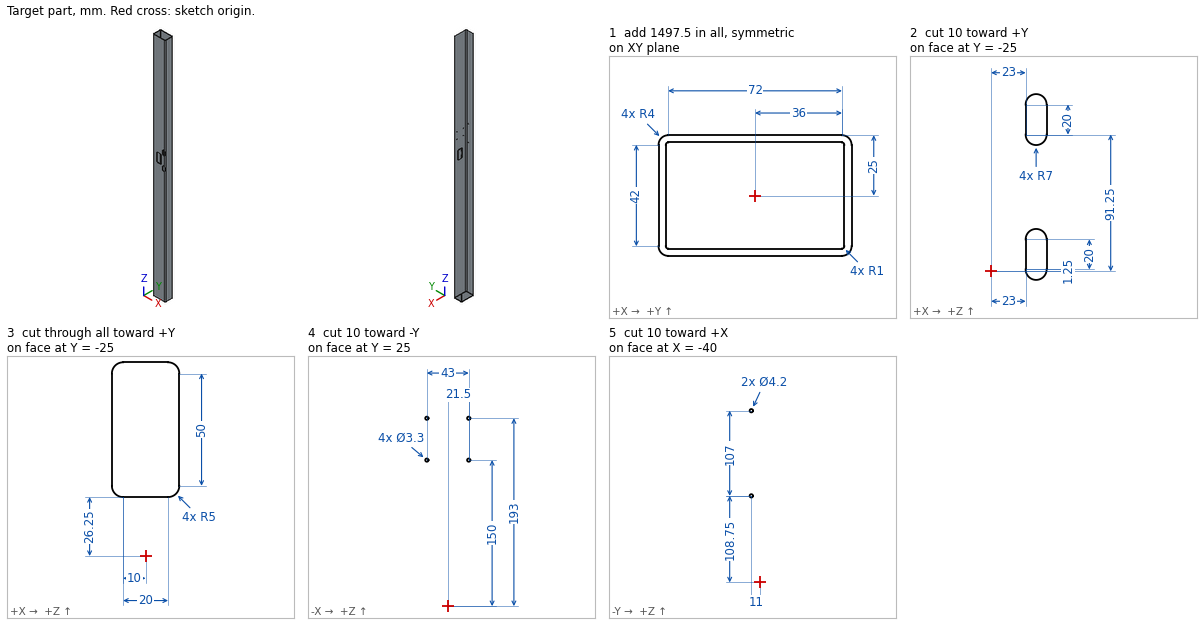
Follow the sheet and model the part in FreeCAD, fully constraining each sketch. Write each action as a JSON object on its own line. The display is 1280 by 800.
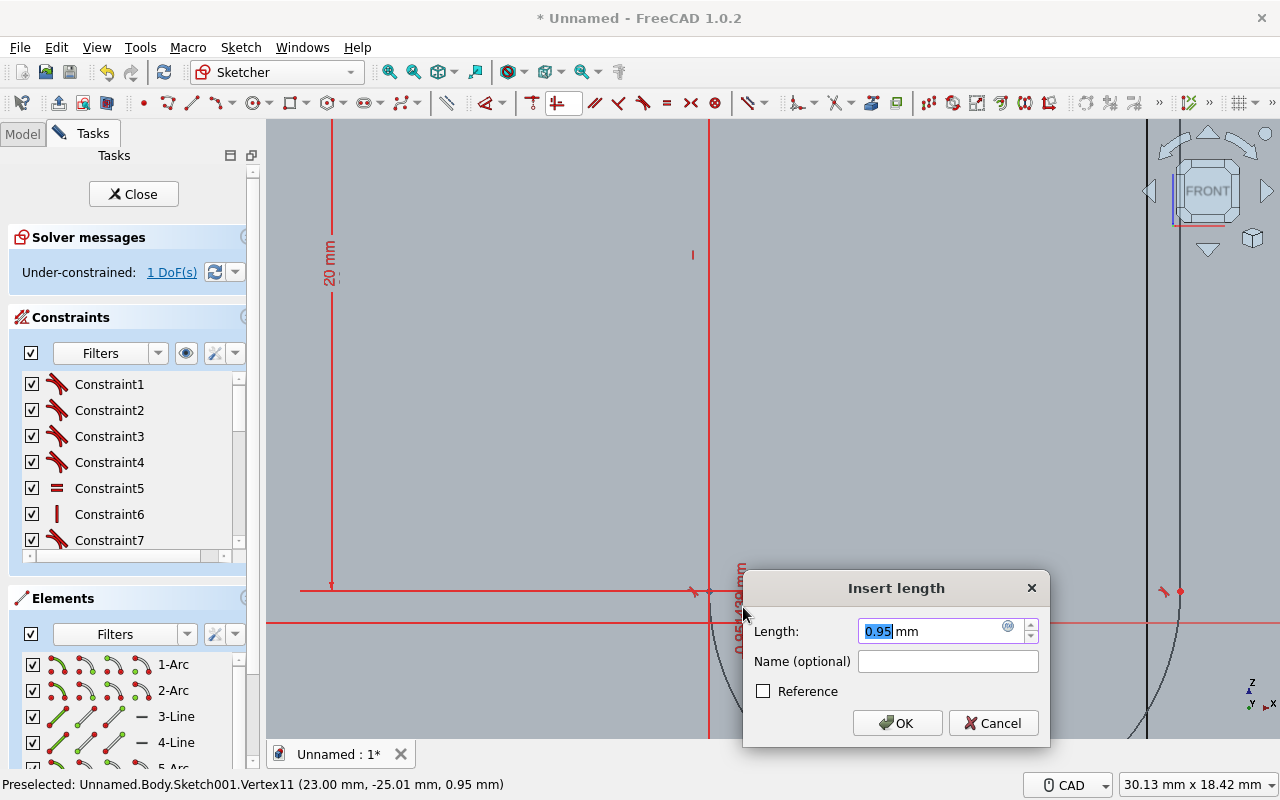
{"action": "type", "text": "1.25"}
{"action": "key", "text": "Return"}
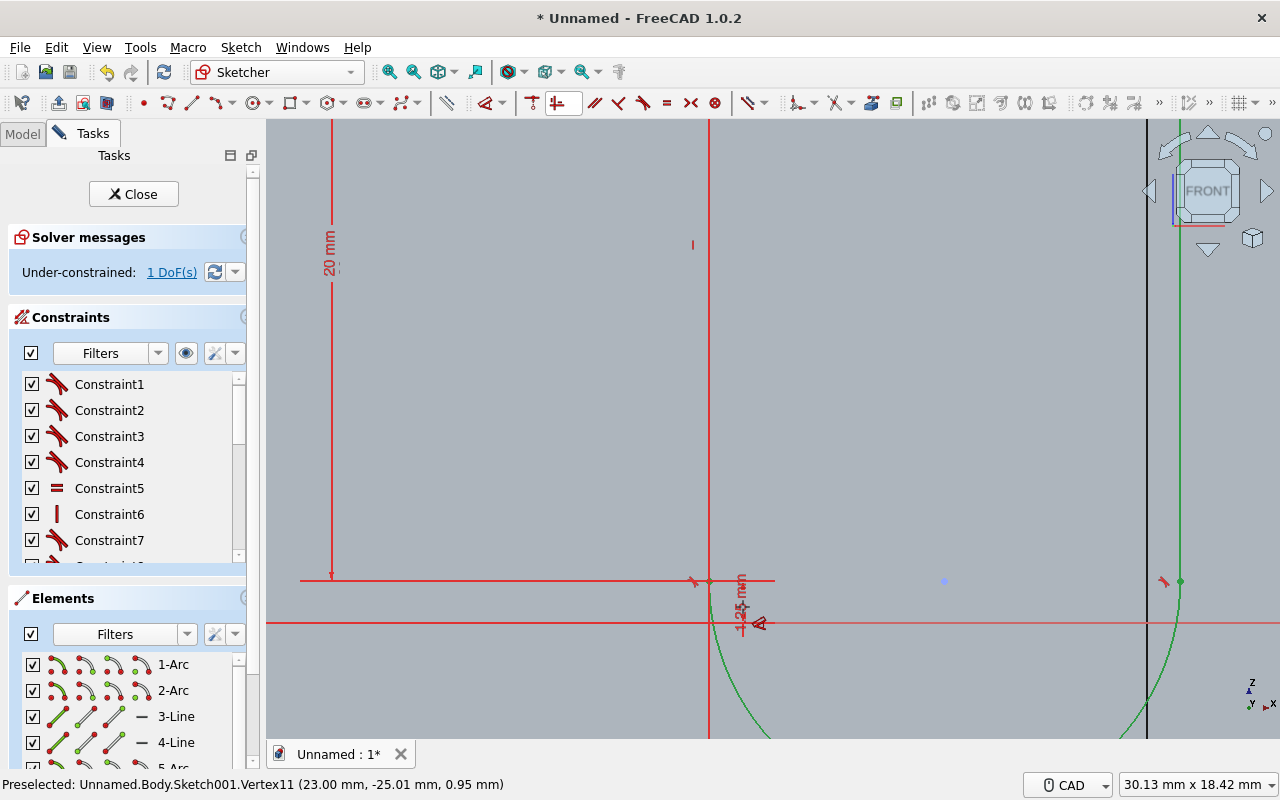
{"action": "scroll", "coordinate": [719, 599], "scroll_direction": "down", "scroll_amount": 12}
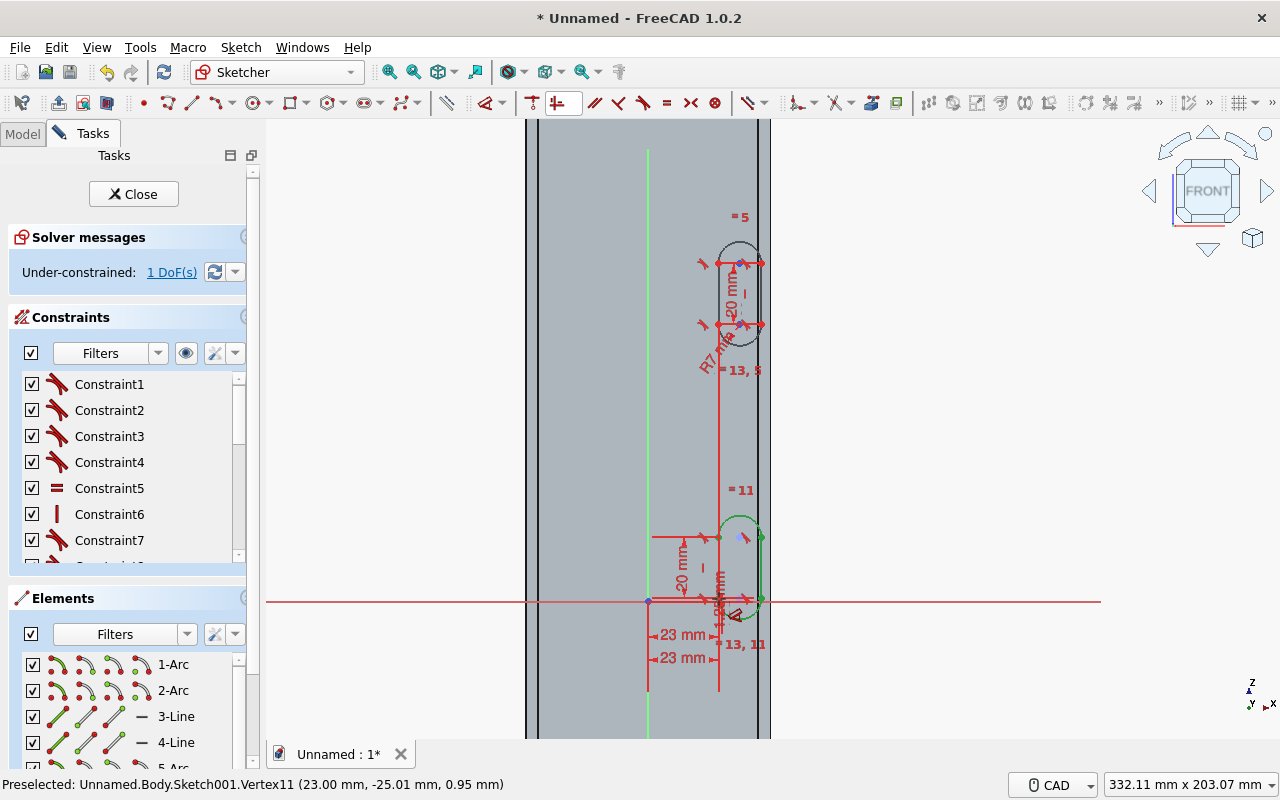
{"action": "left_click", "coordinate": [719, 324]}
{"action": "left_click", "coordinate": [614, 463]}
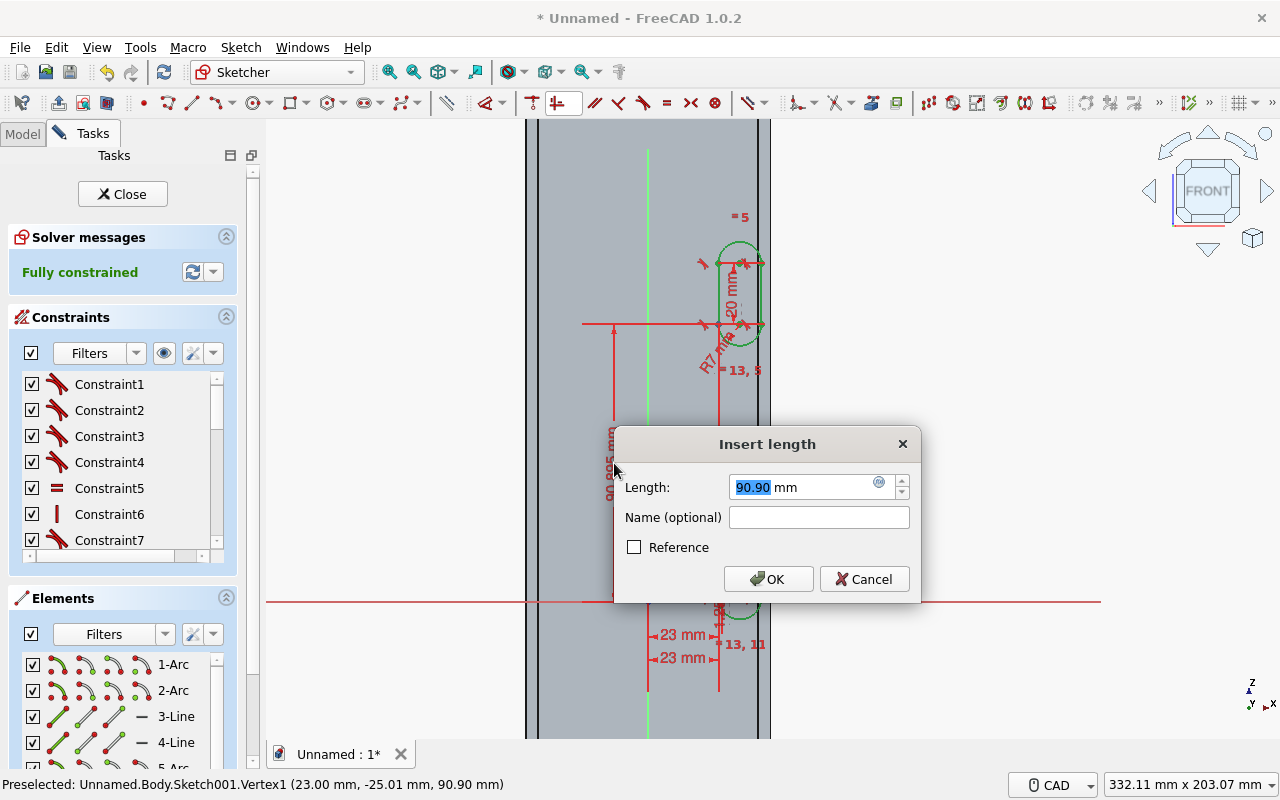
{"action": "type", "text": "91.25"}
{"action": "key", "text": "Return"}
{"action": "key", "text": "Escape"}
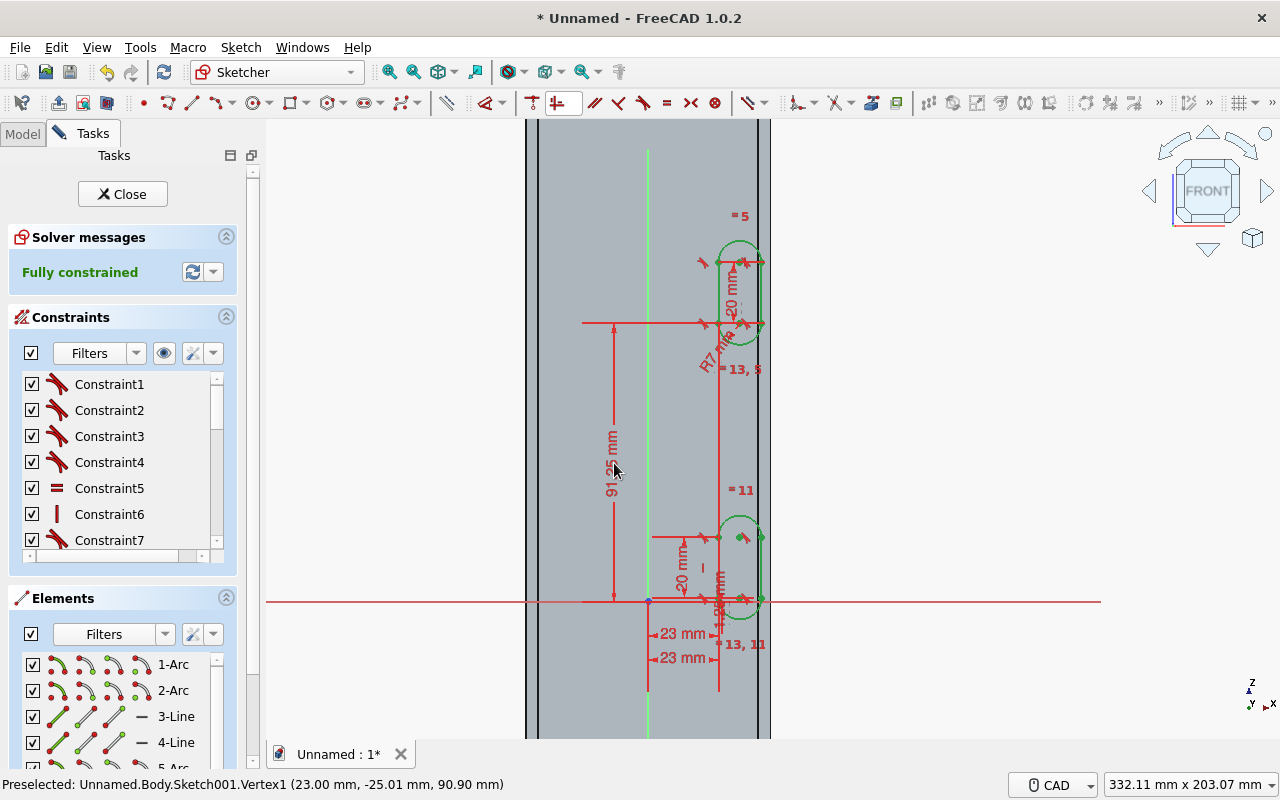
{"action": "left_click", "coordinate": [123, 194]}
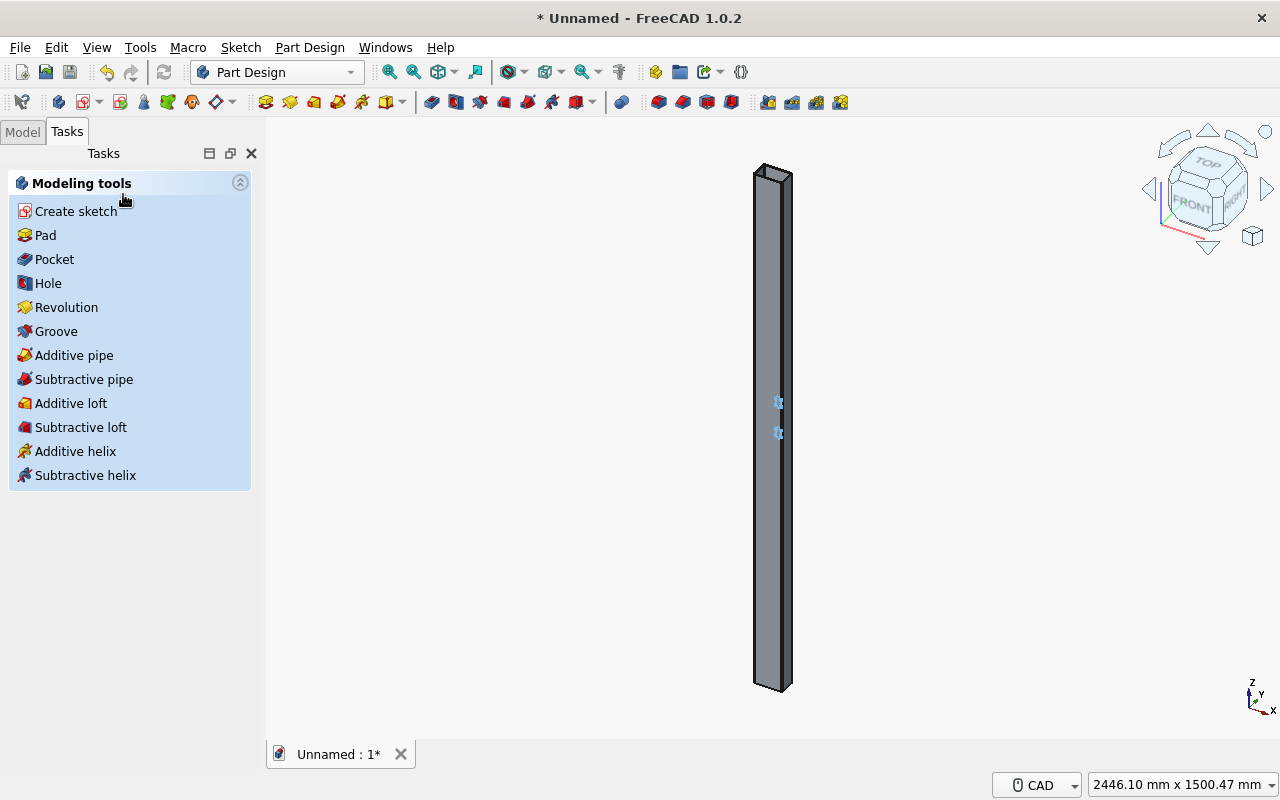
{"action": "left_click", "coordinate": [432, 102]}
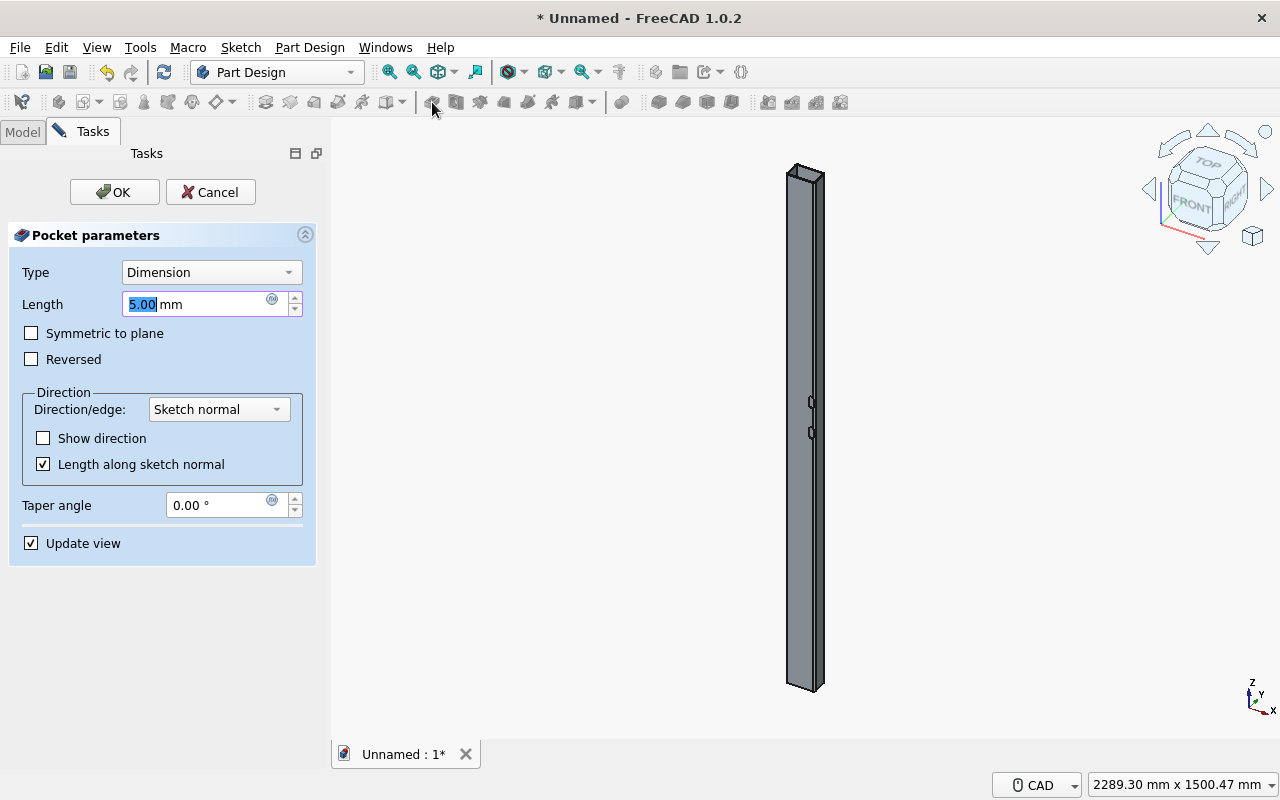
{"action": "type", "text": "10"}
{"action": "key", "text": "Tab"}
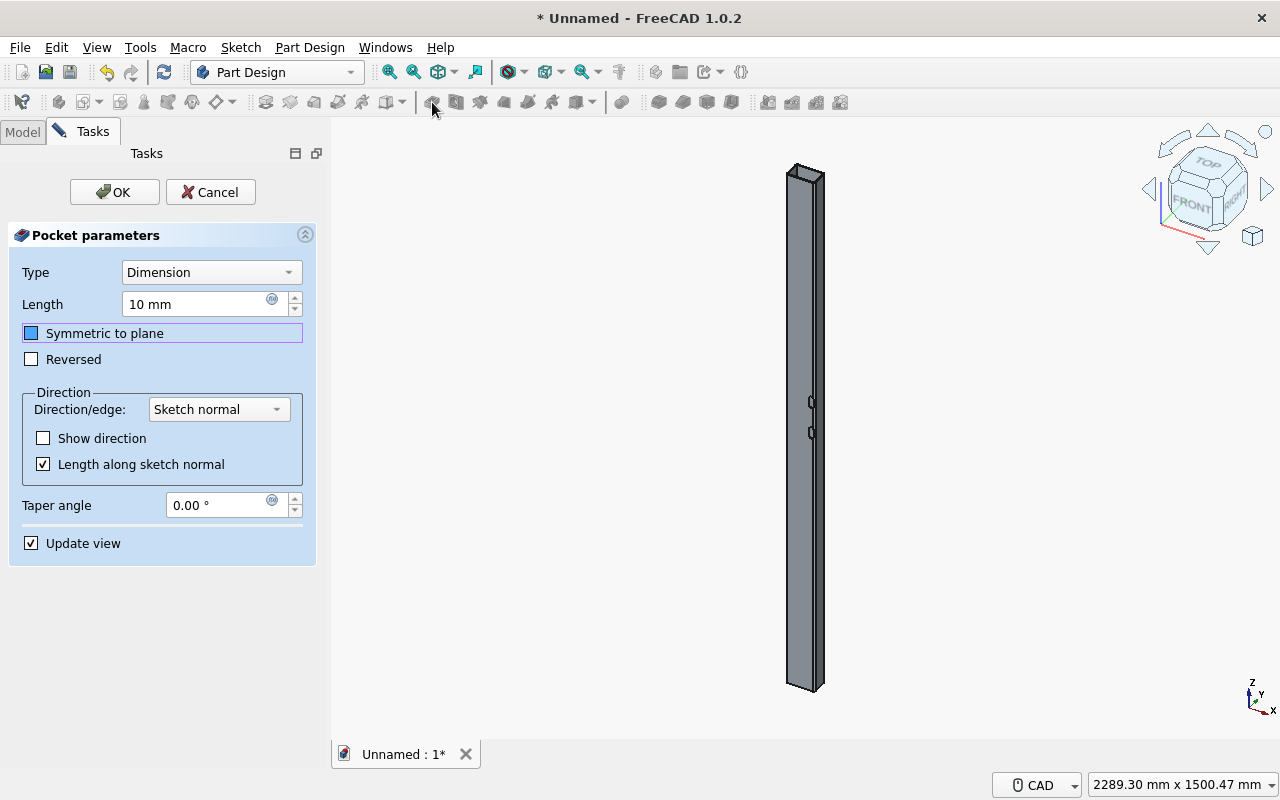
{"action": "left_click", "coordinate": [115, 192]}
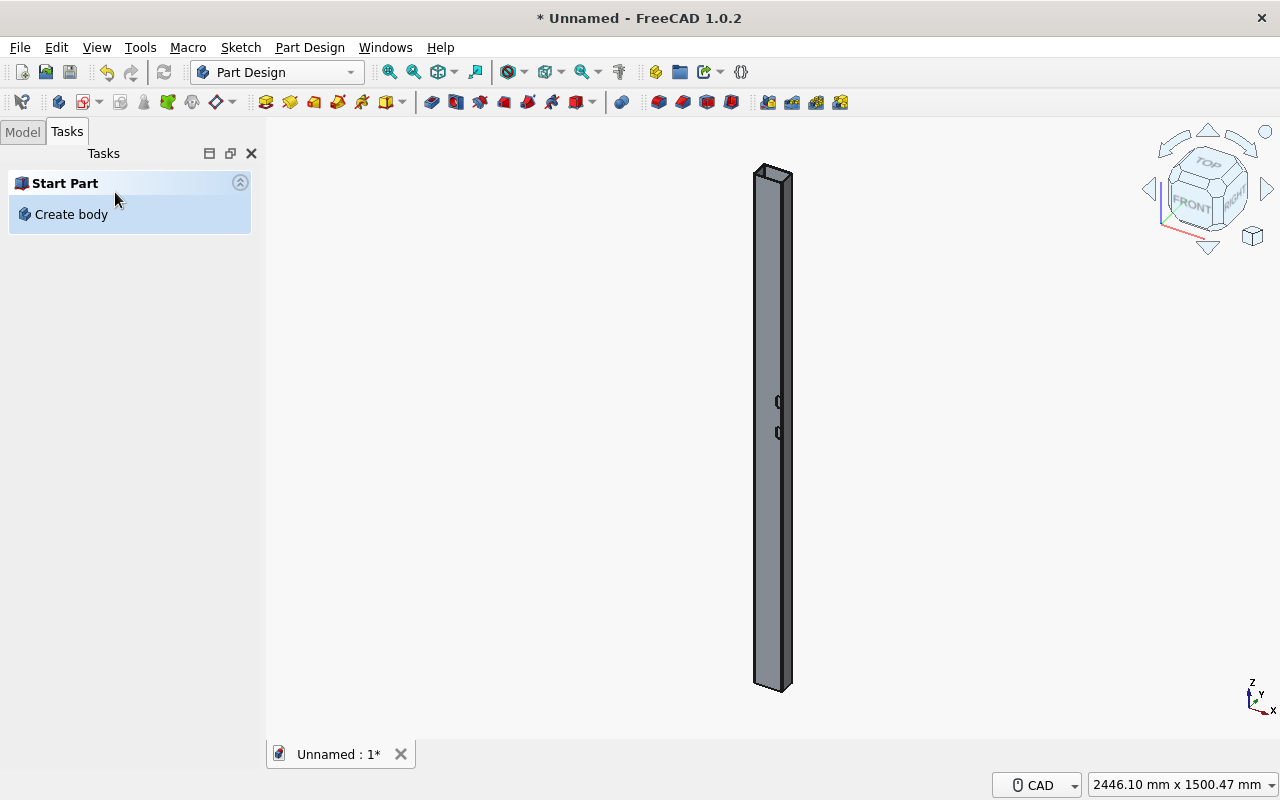
{"action": "left_click", "coordinate": [768, 214]}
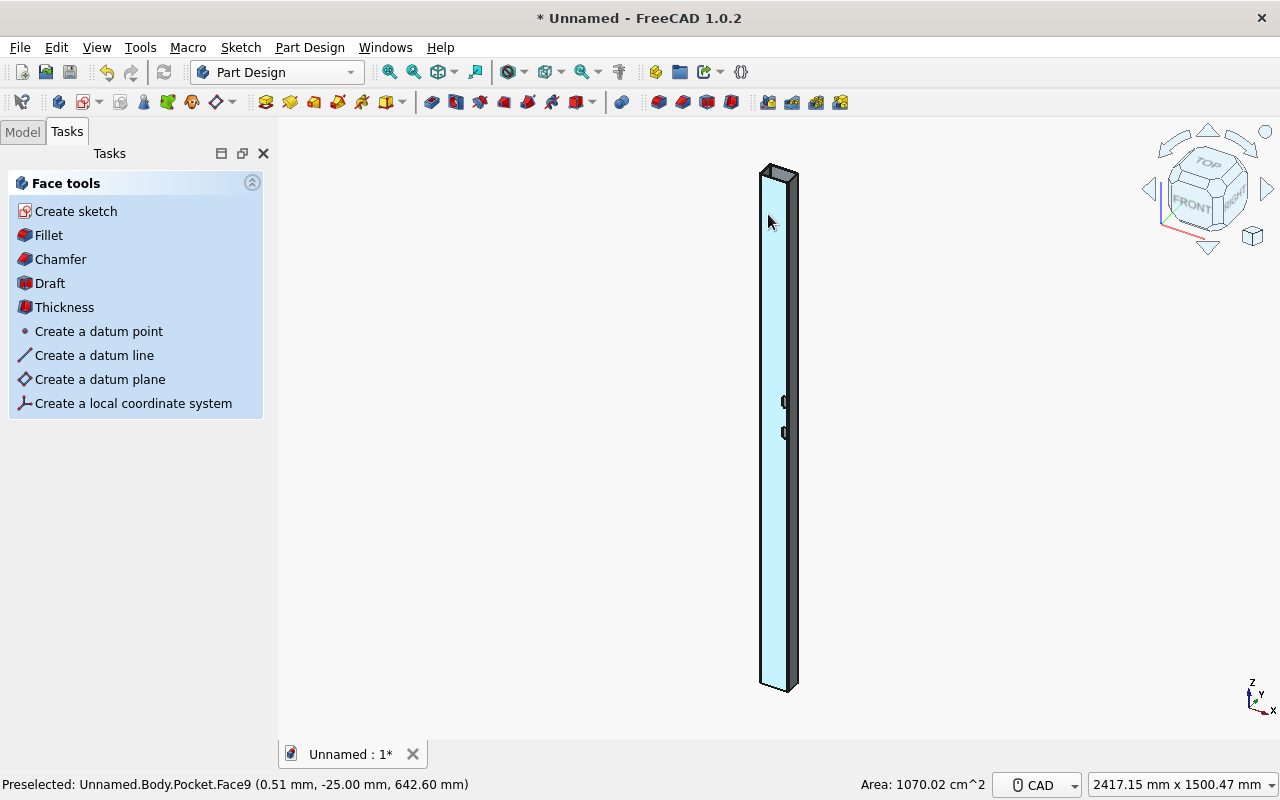
{"action": "left_click", "coordinate": [84, 102]}